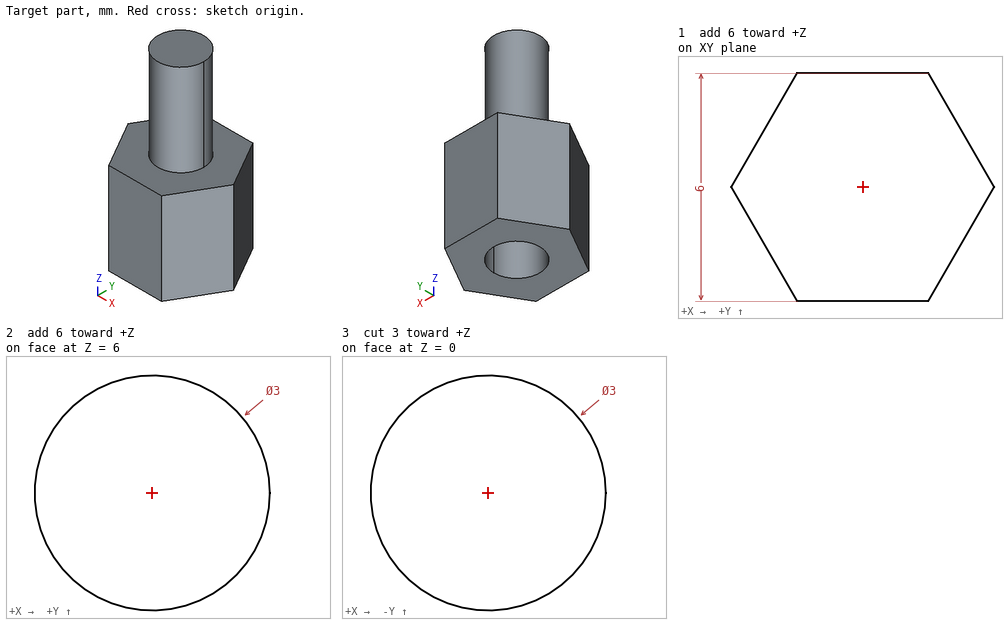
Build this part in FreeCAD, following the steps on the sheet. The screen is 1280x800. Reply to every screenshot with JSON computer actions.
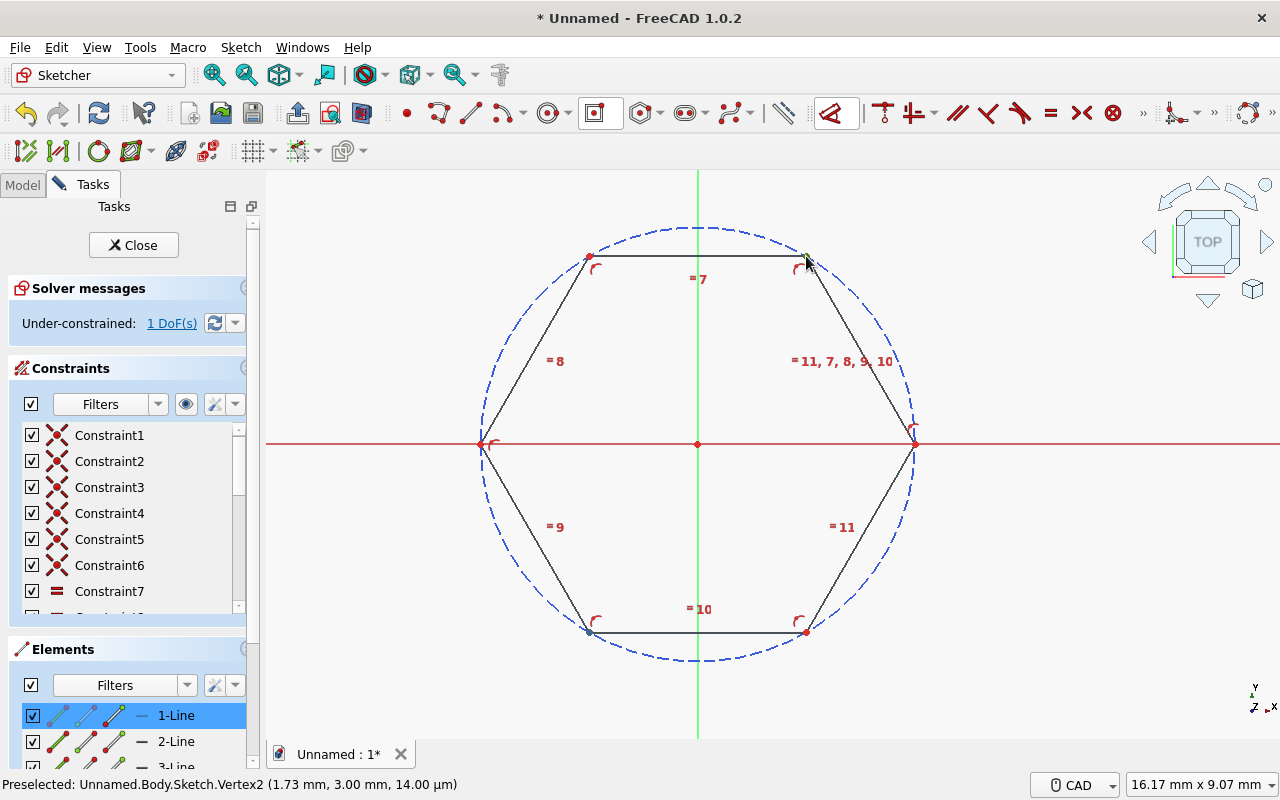
{"action": "left_click", "coordinate": [854, 114]}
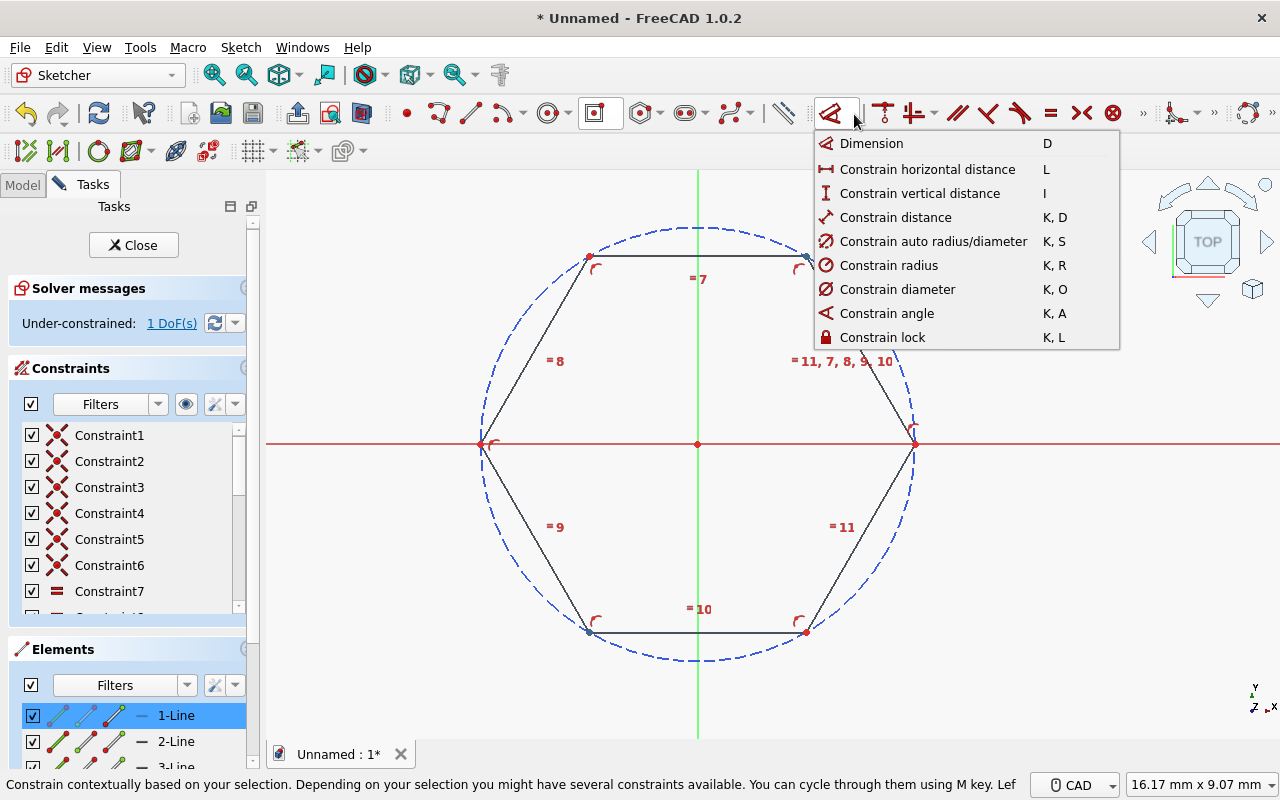
{"action": "left_click", "coordinate": [967, 193]}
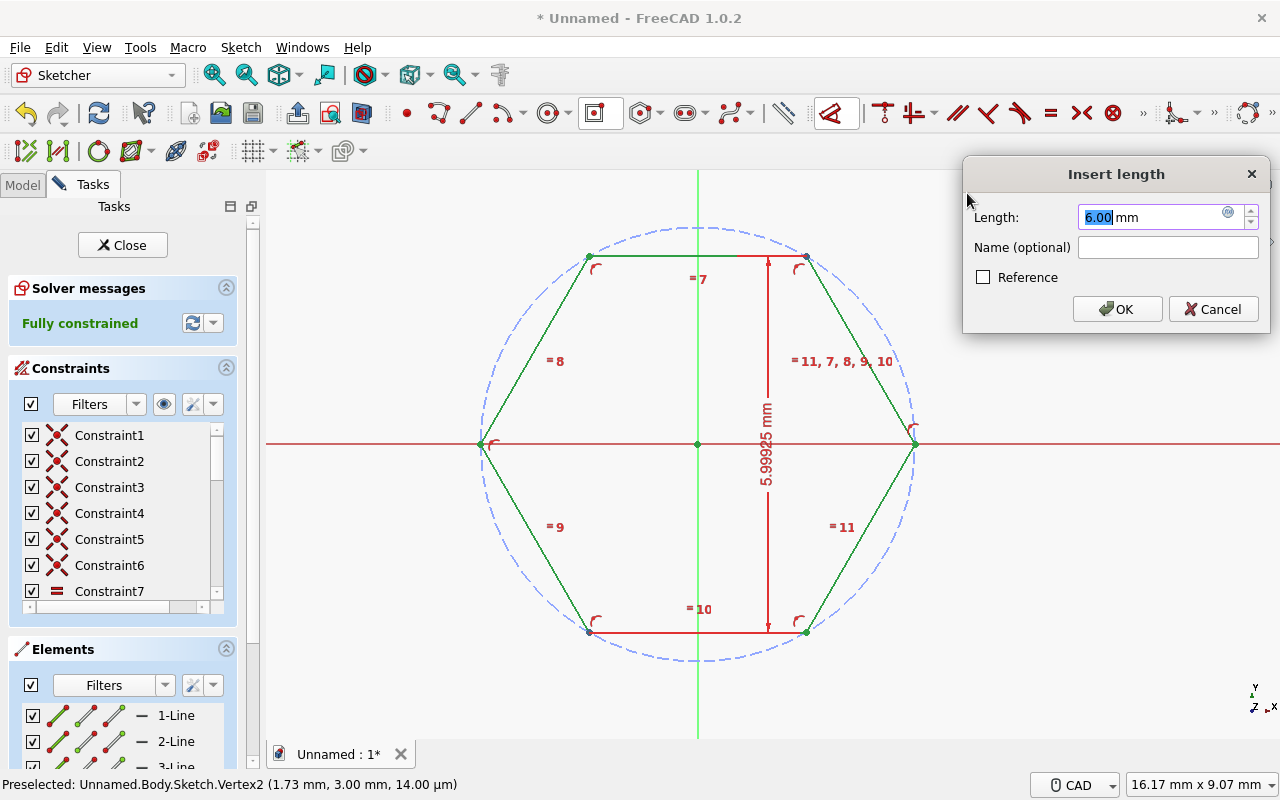
{"action": "type", "text": "6"}
{"action": "key", "text": "Return"}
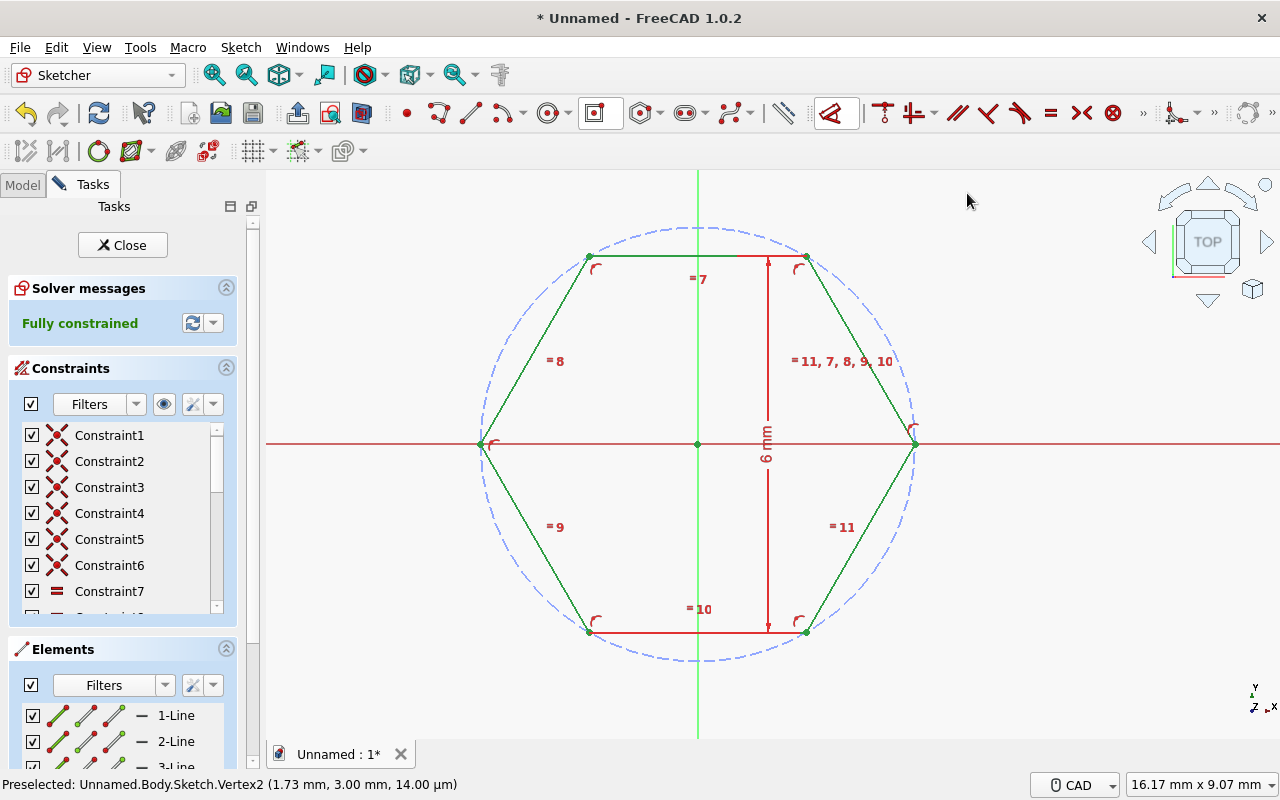
{"action": "left_click", "coordinate": [123, 245]}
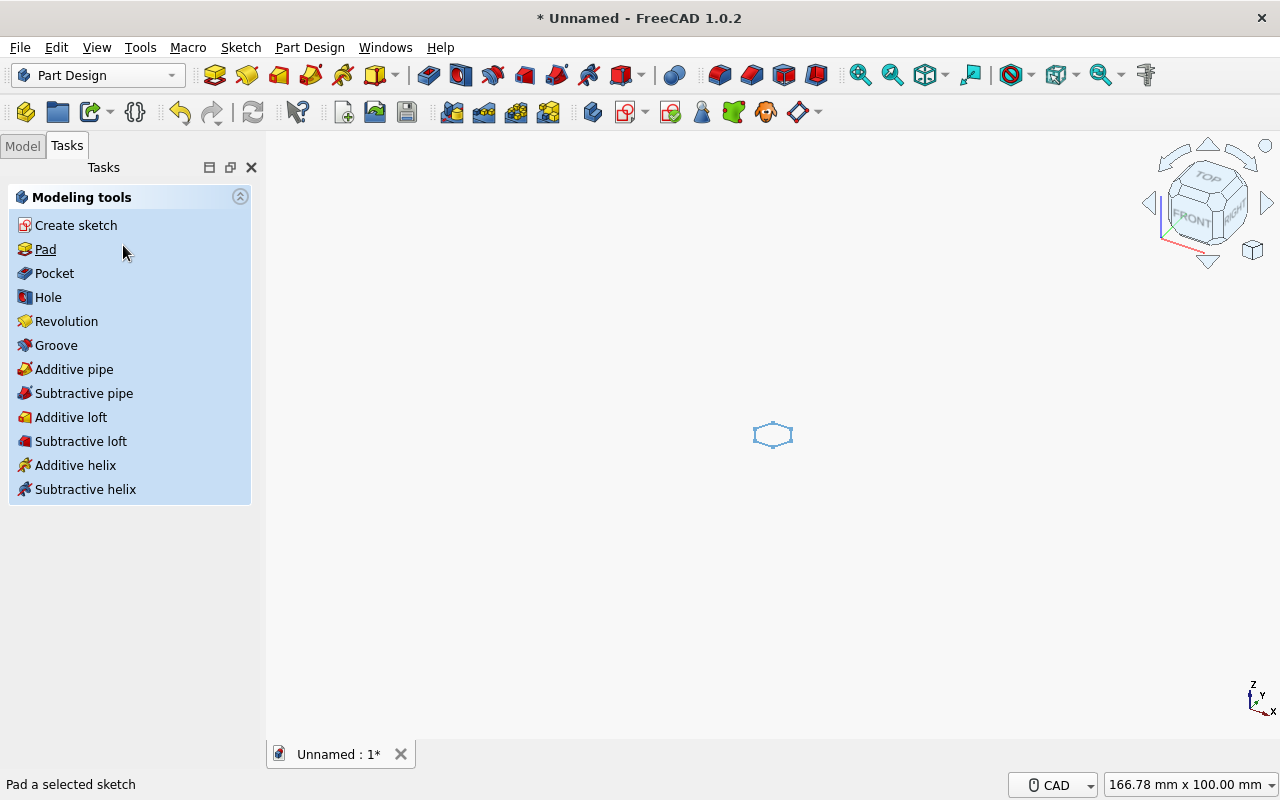
{"action": "left_click", "coordinate": [216, 76]}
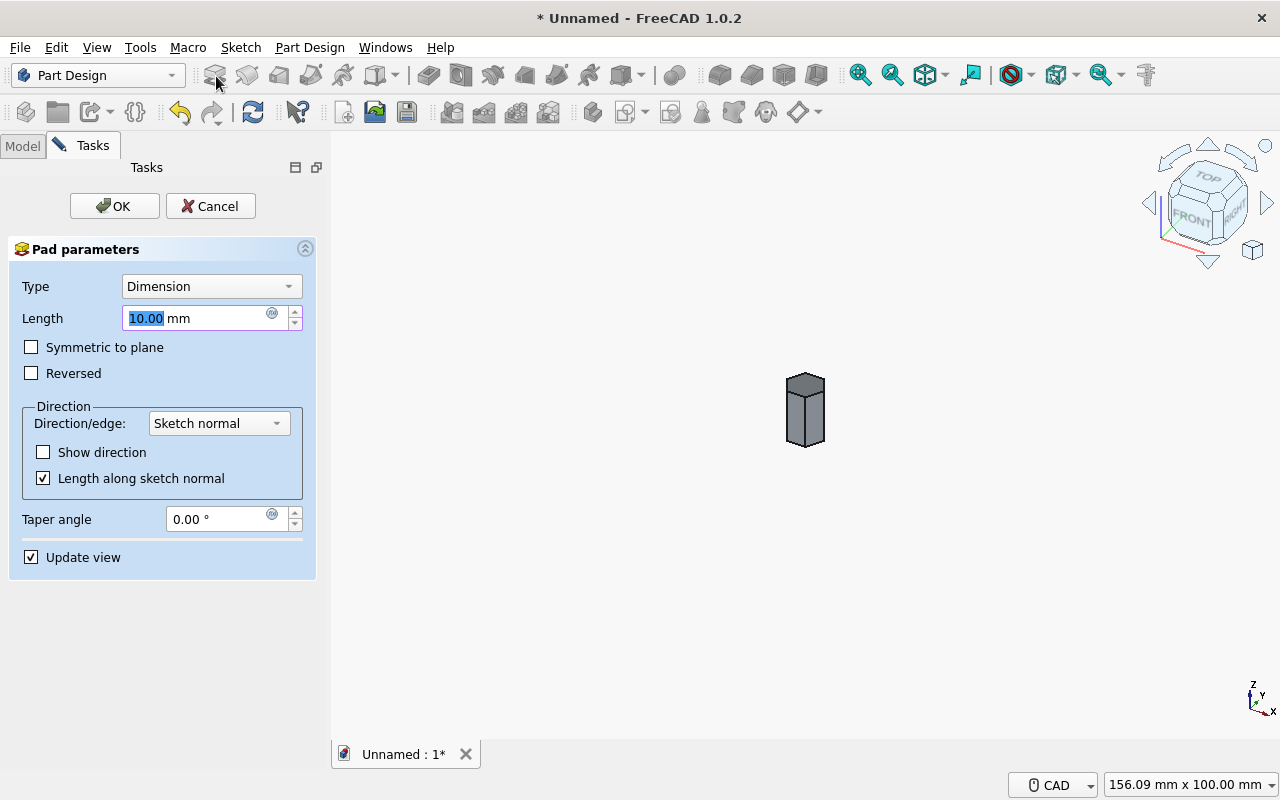
{"action": "type", "text": "6"}
{"action": "key", "text": "Tab"}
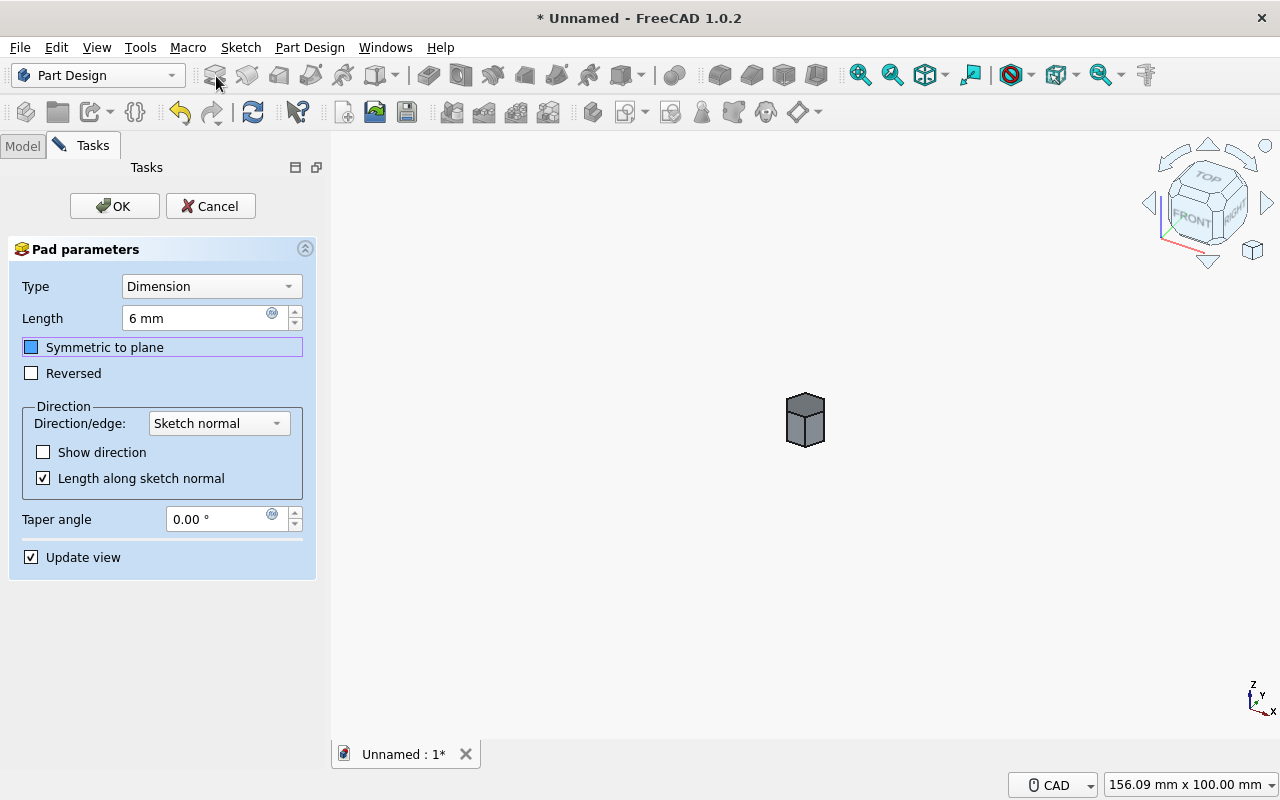
{"action": "left_click", "coordinate": [115, 206]}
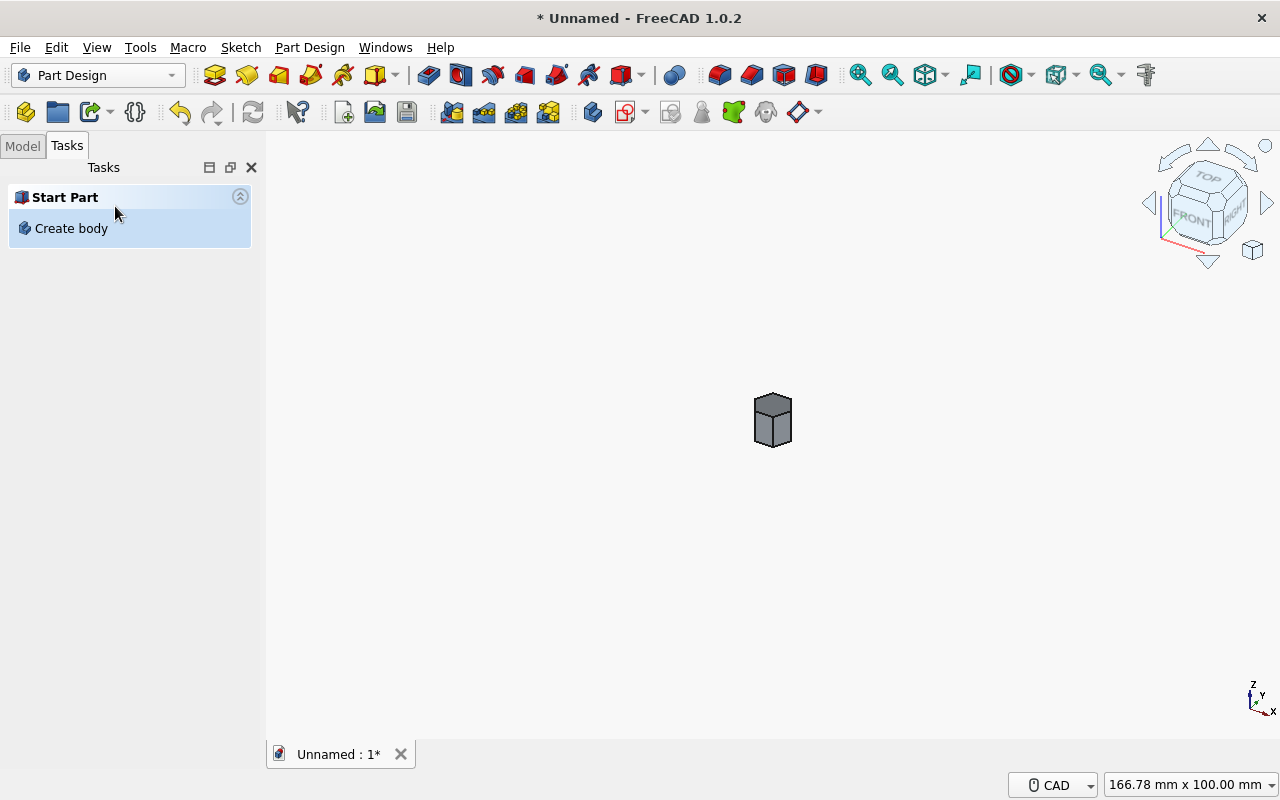
{"action": "left_click", "coordinate": [862, 76]}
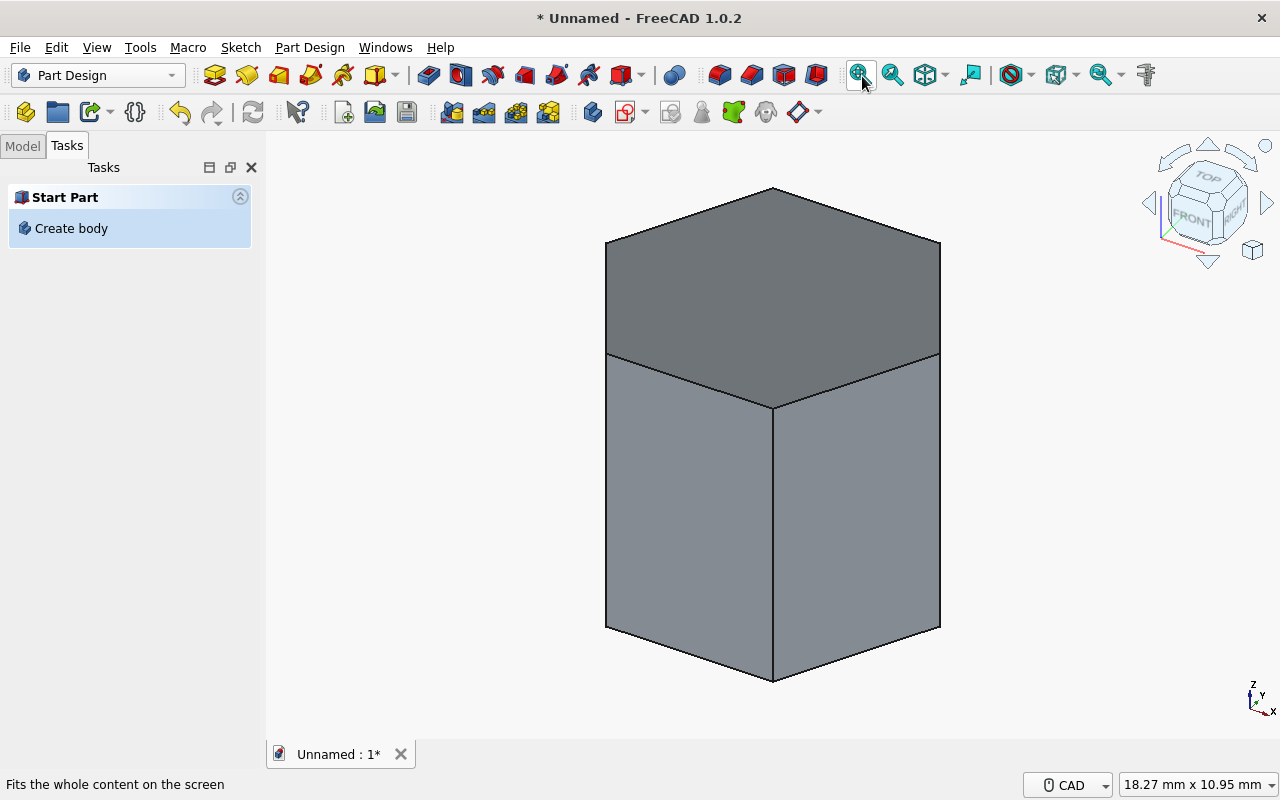
{"action": "left_click", "coordinate": [773, 298]}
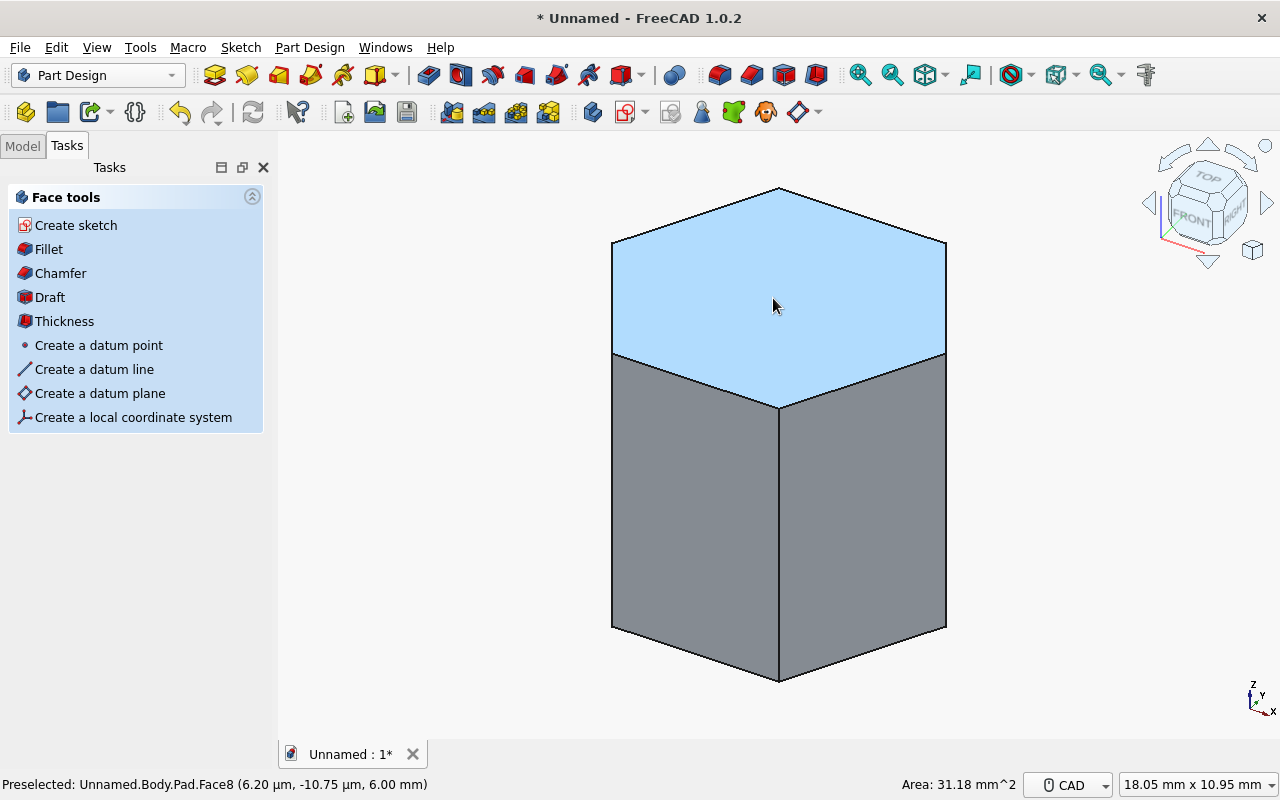
{"action": "left_click", "coordinate": [626, 112]}